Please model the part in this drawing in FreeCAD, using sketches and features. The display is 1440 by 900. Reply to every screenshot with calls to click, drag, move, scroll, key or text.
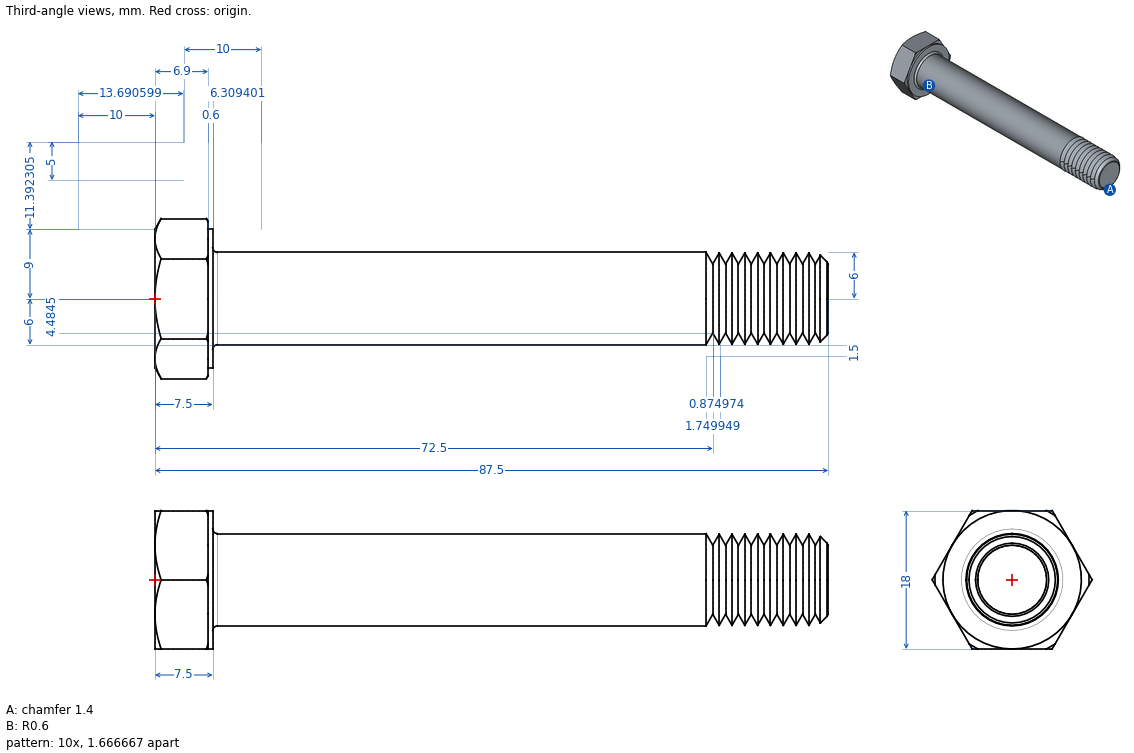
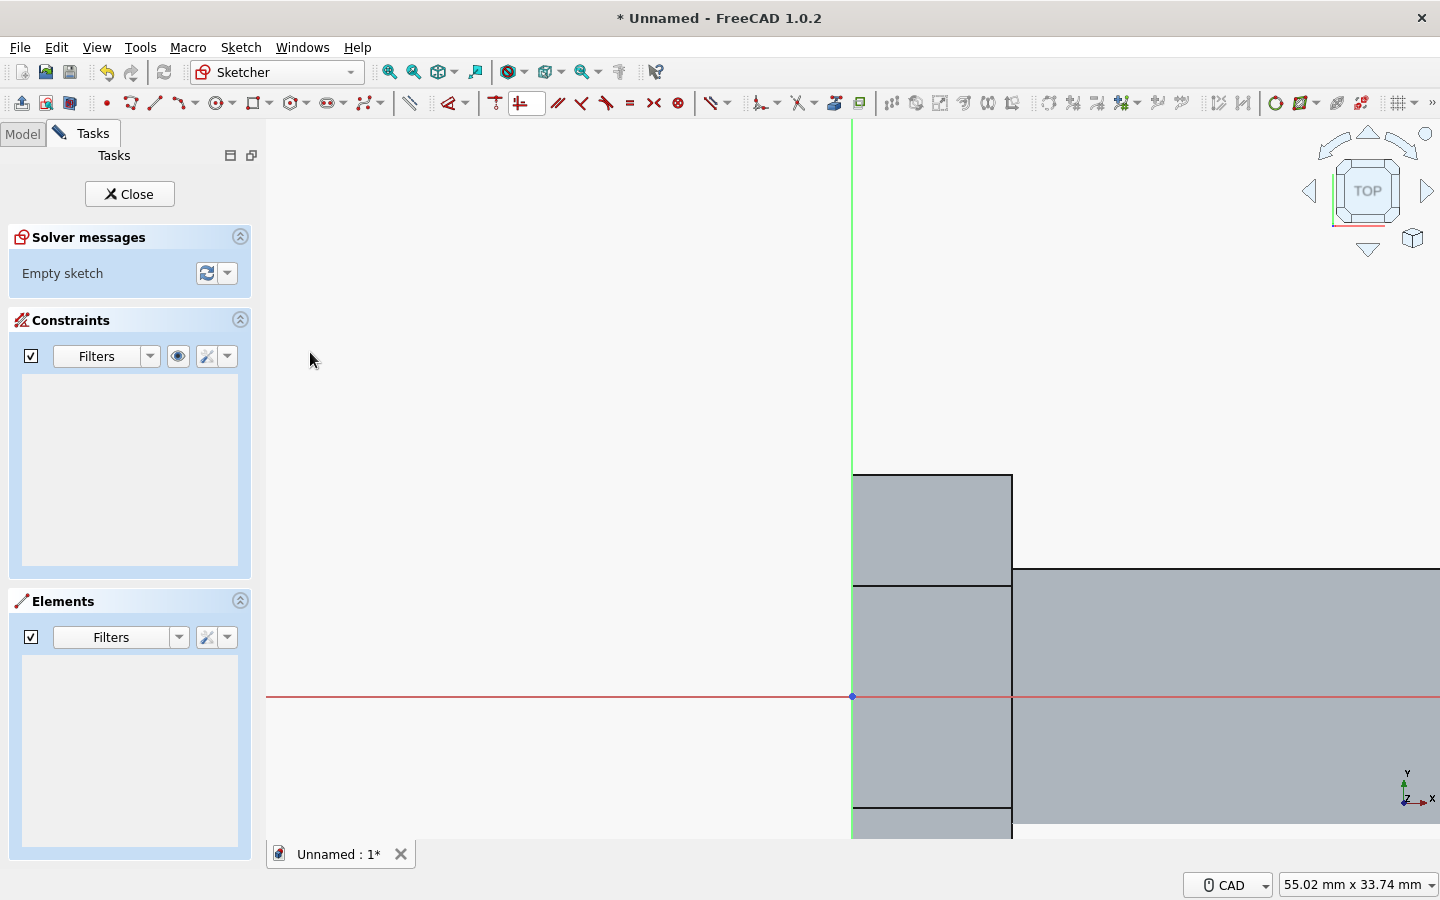
click(132, 104)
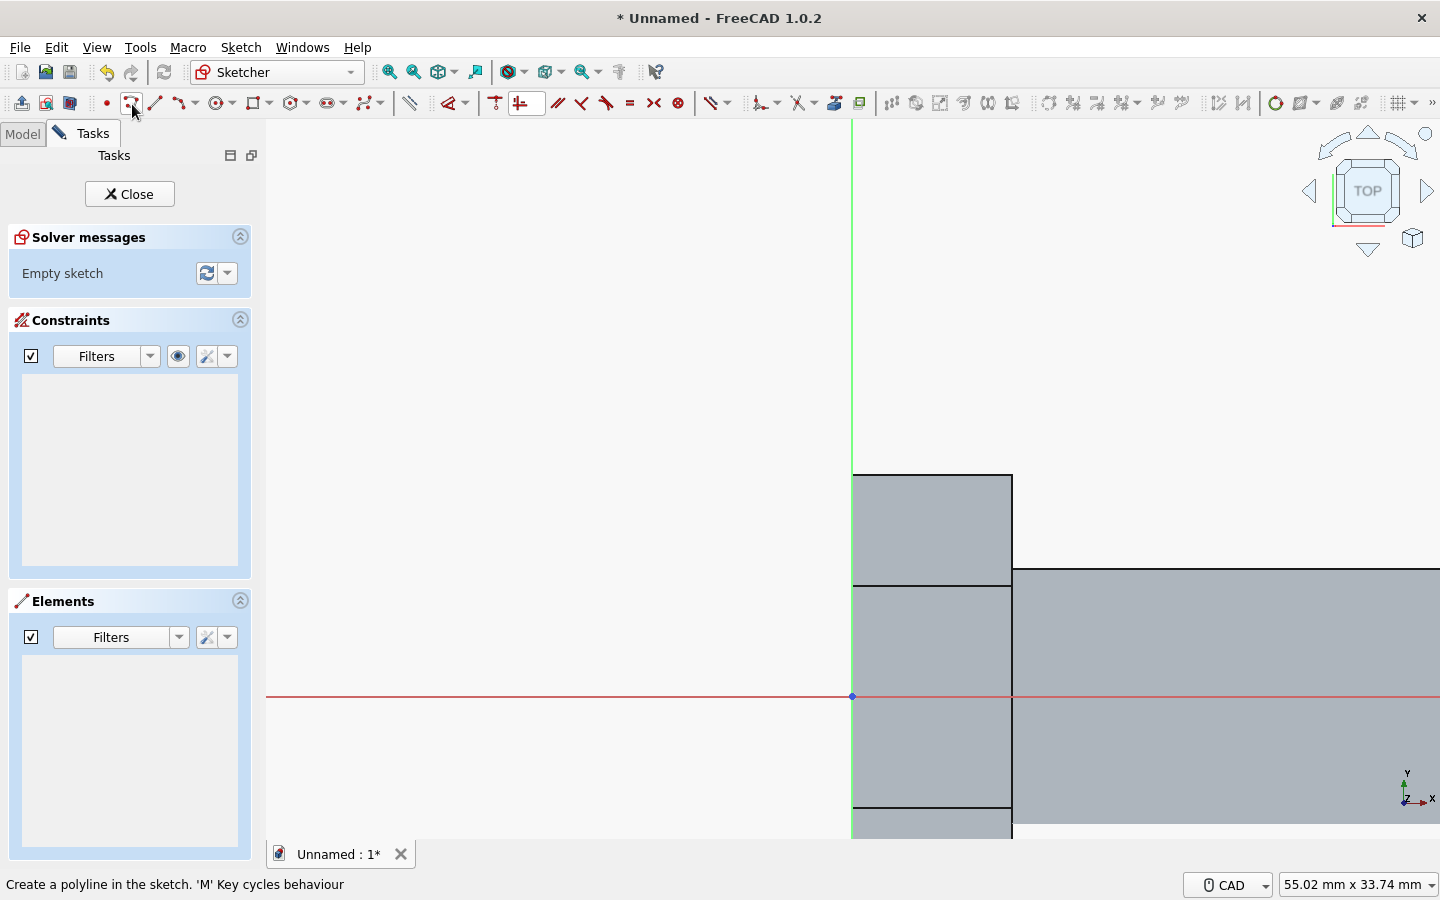
click(852, 505)
click(931, 368)
click(931, 262)
click(639, 262)
click(639, 505)
click(852, 506)
key(Escape)
key(Escape)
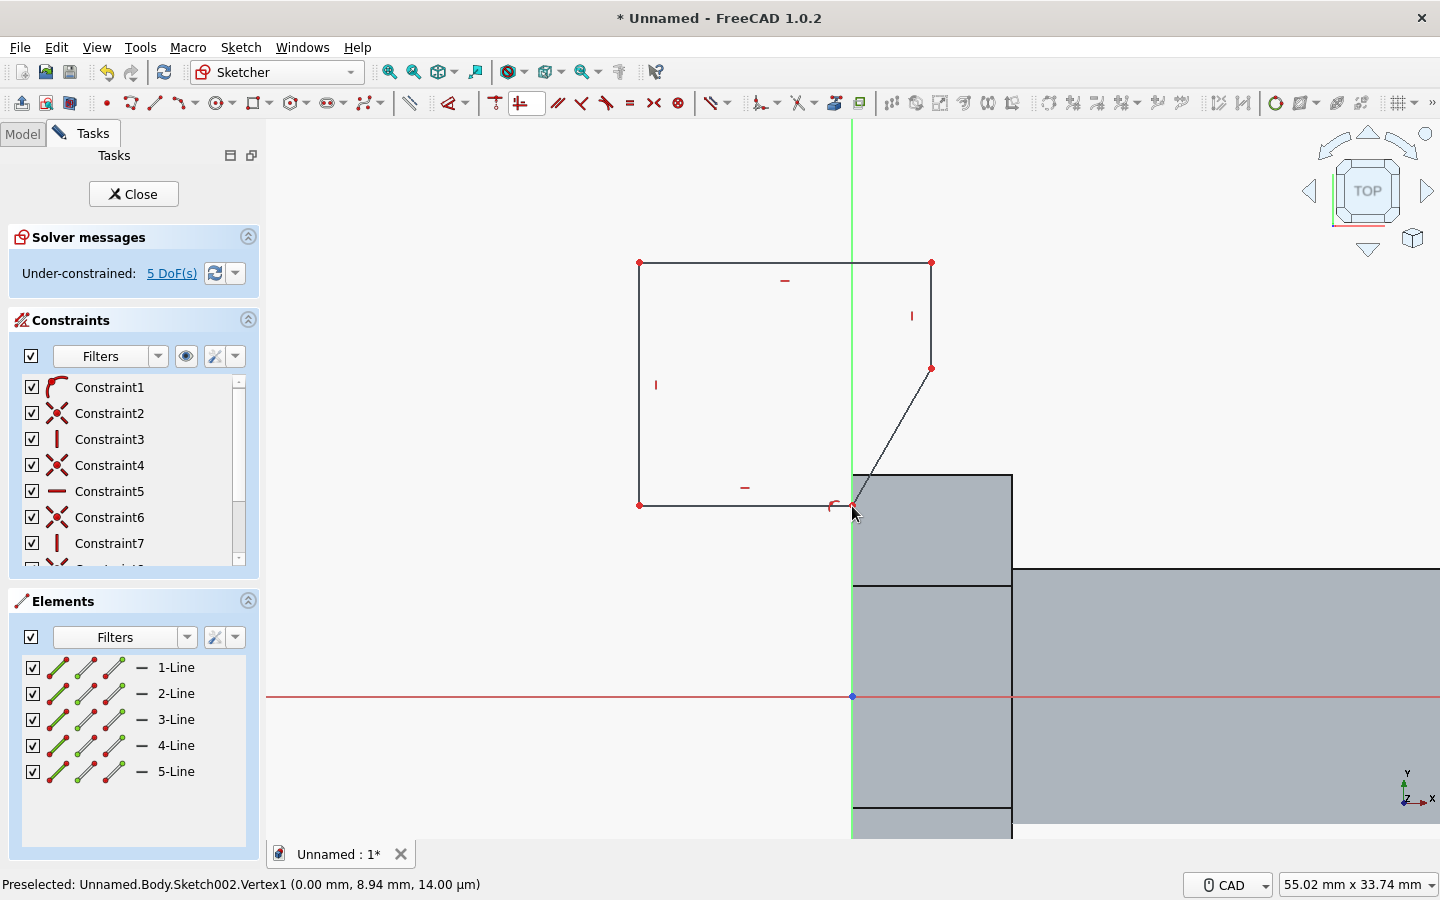
click(448, 104)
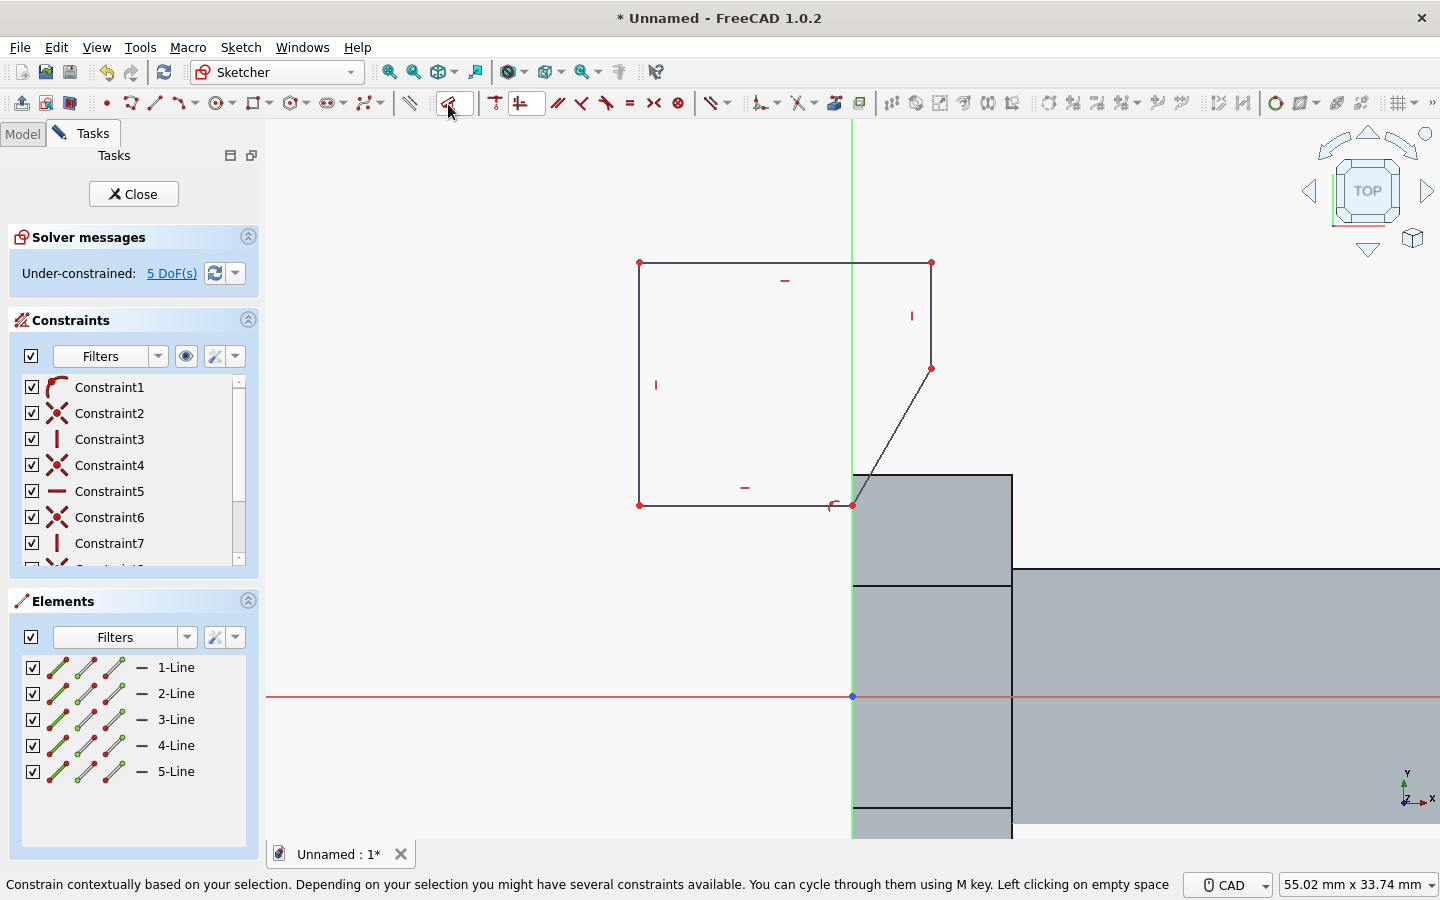
click(931, 337)
click(965, 316)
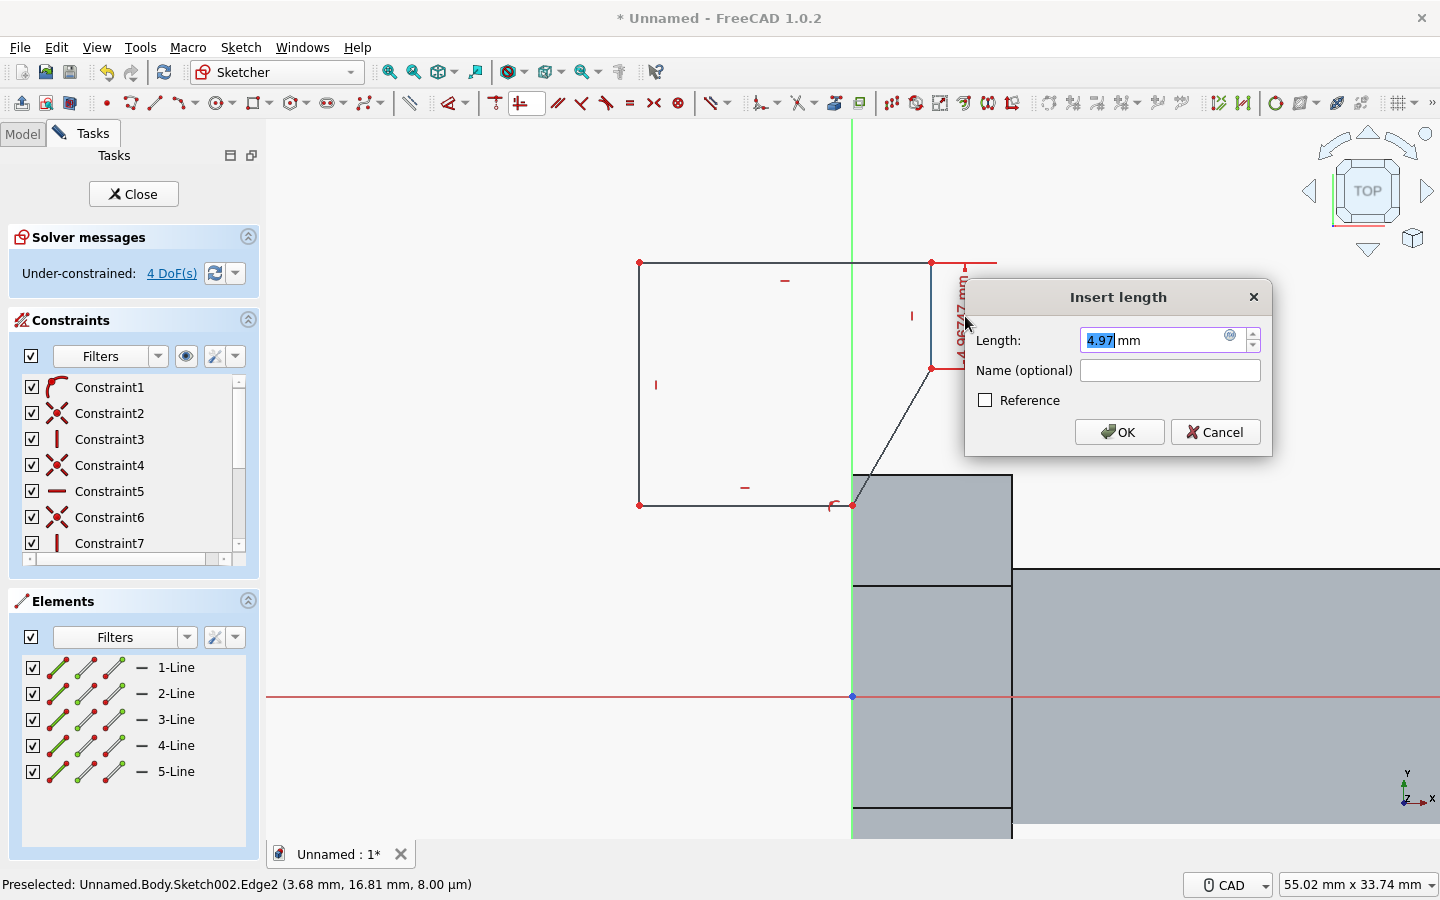
text(5)
key(Return)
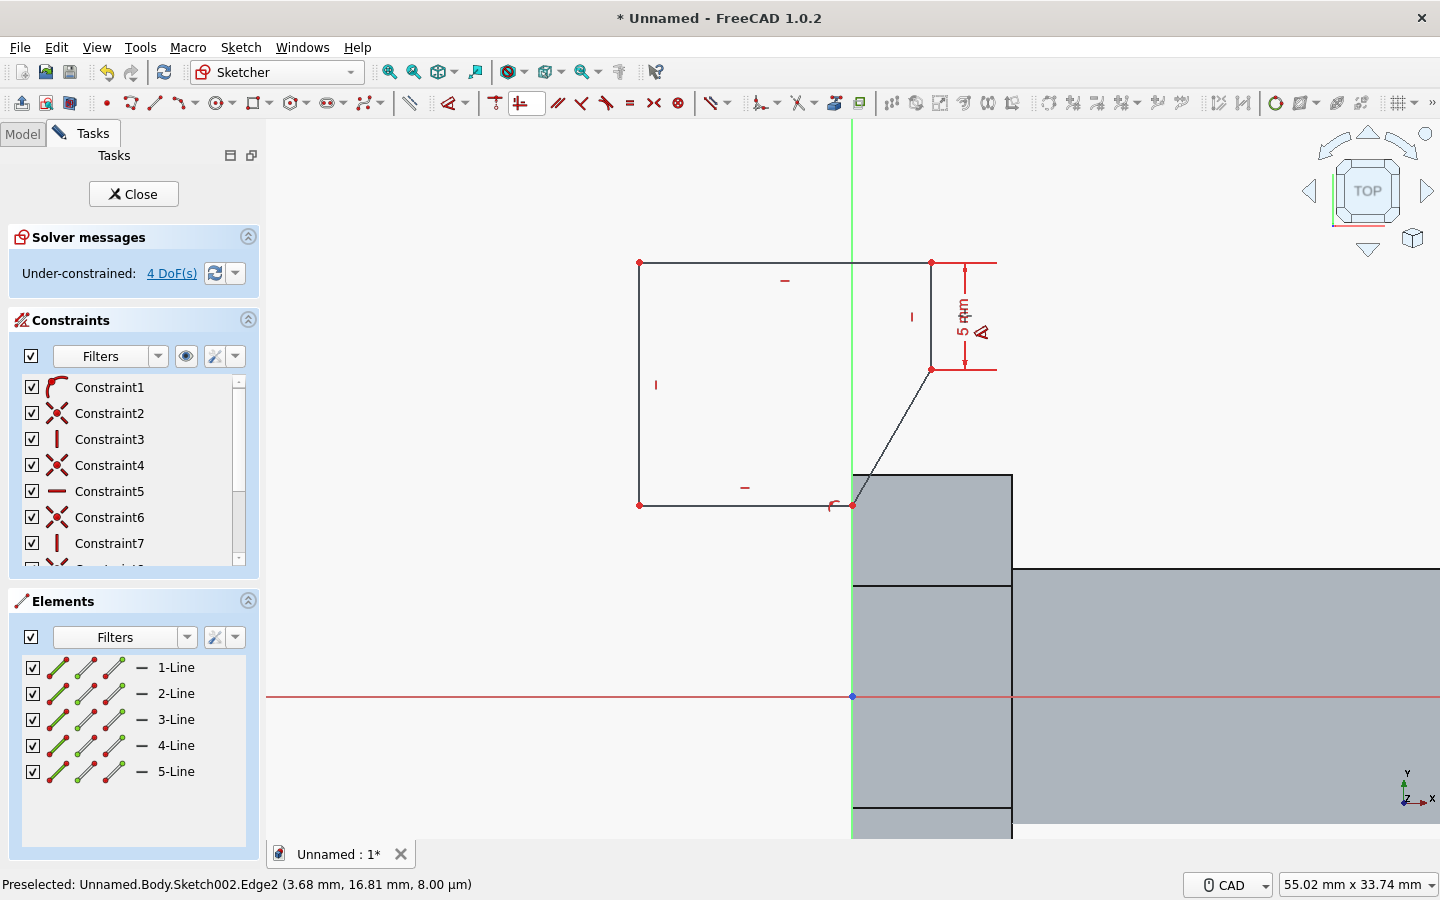
click(703, 506)
click(746, 540)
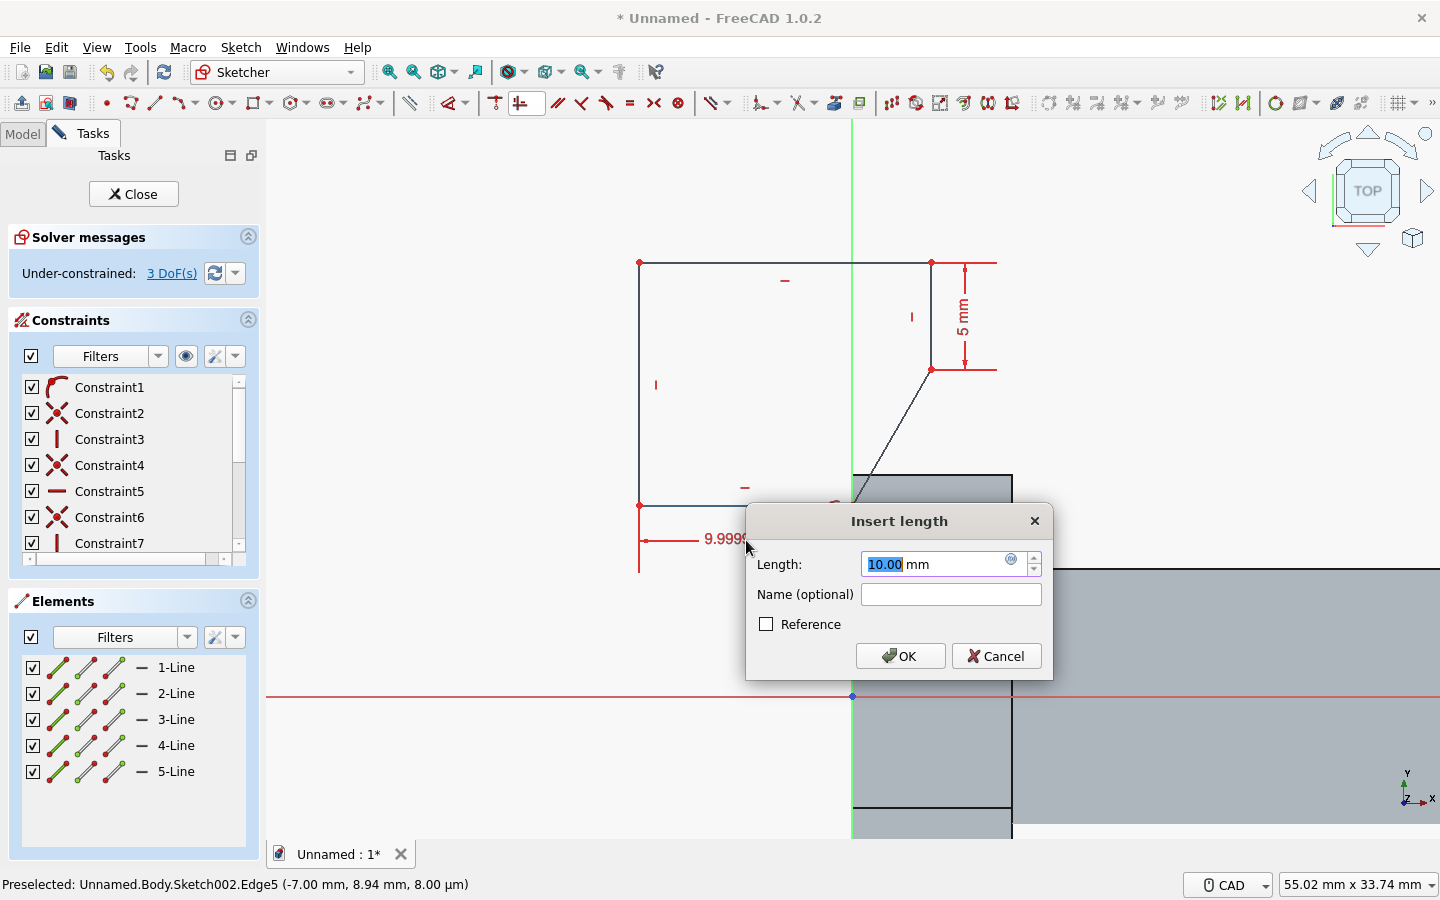
text(10)
key(Return)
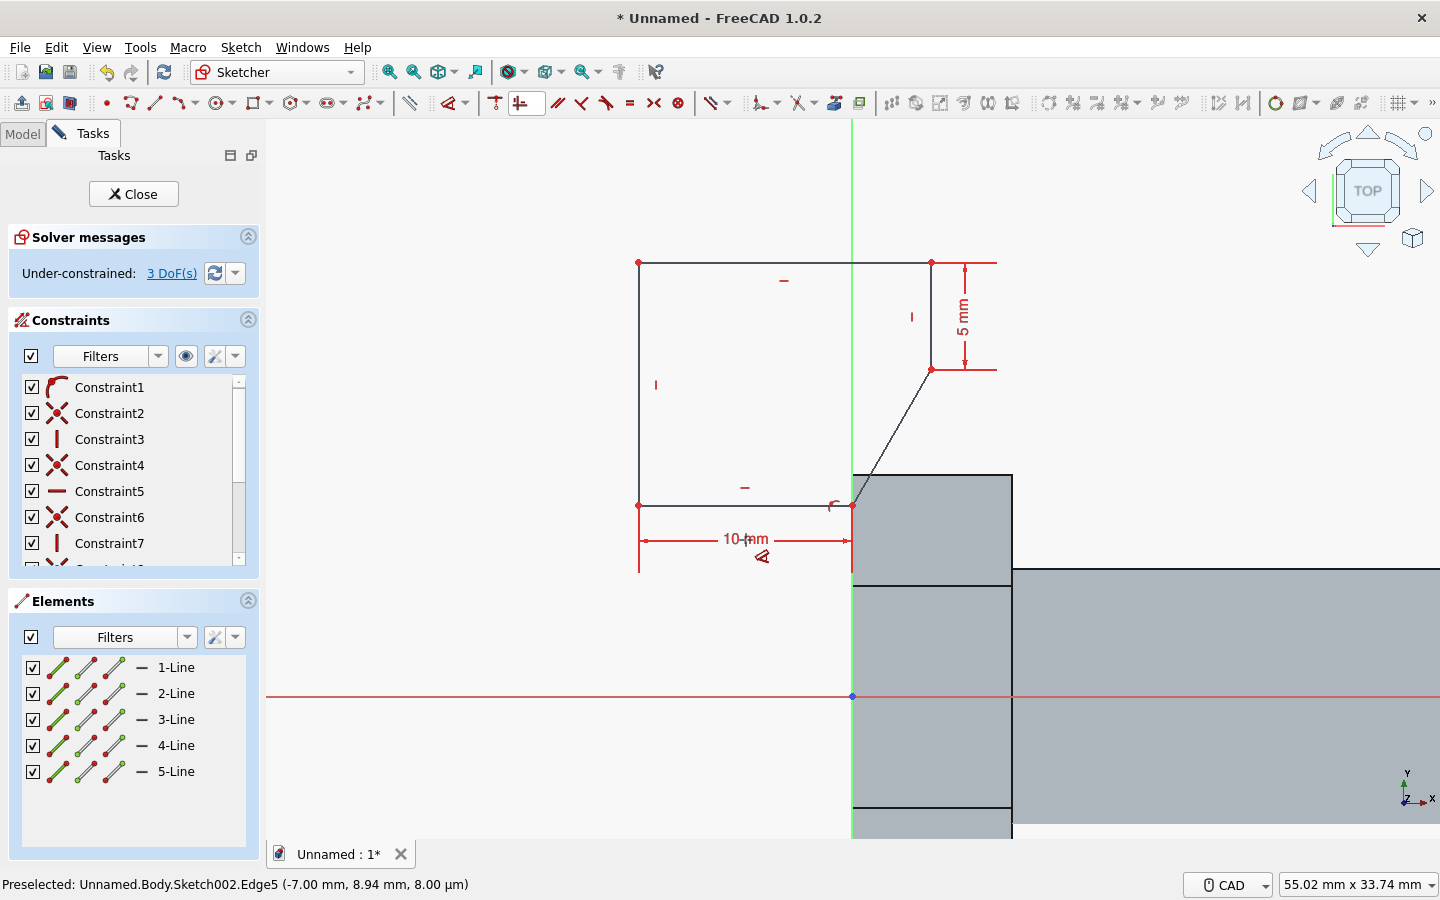
click(852, 506)
click(886, 601)